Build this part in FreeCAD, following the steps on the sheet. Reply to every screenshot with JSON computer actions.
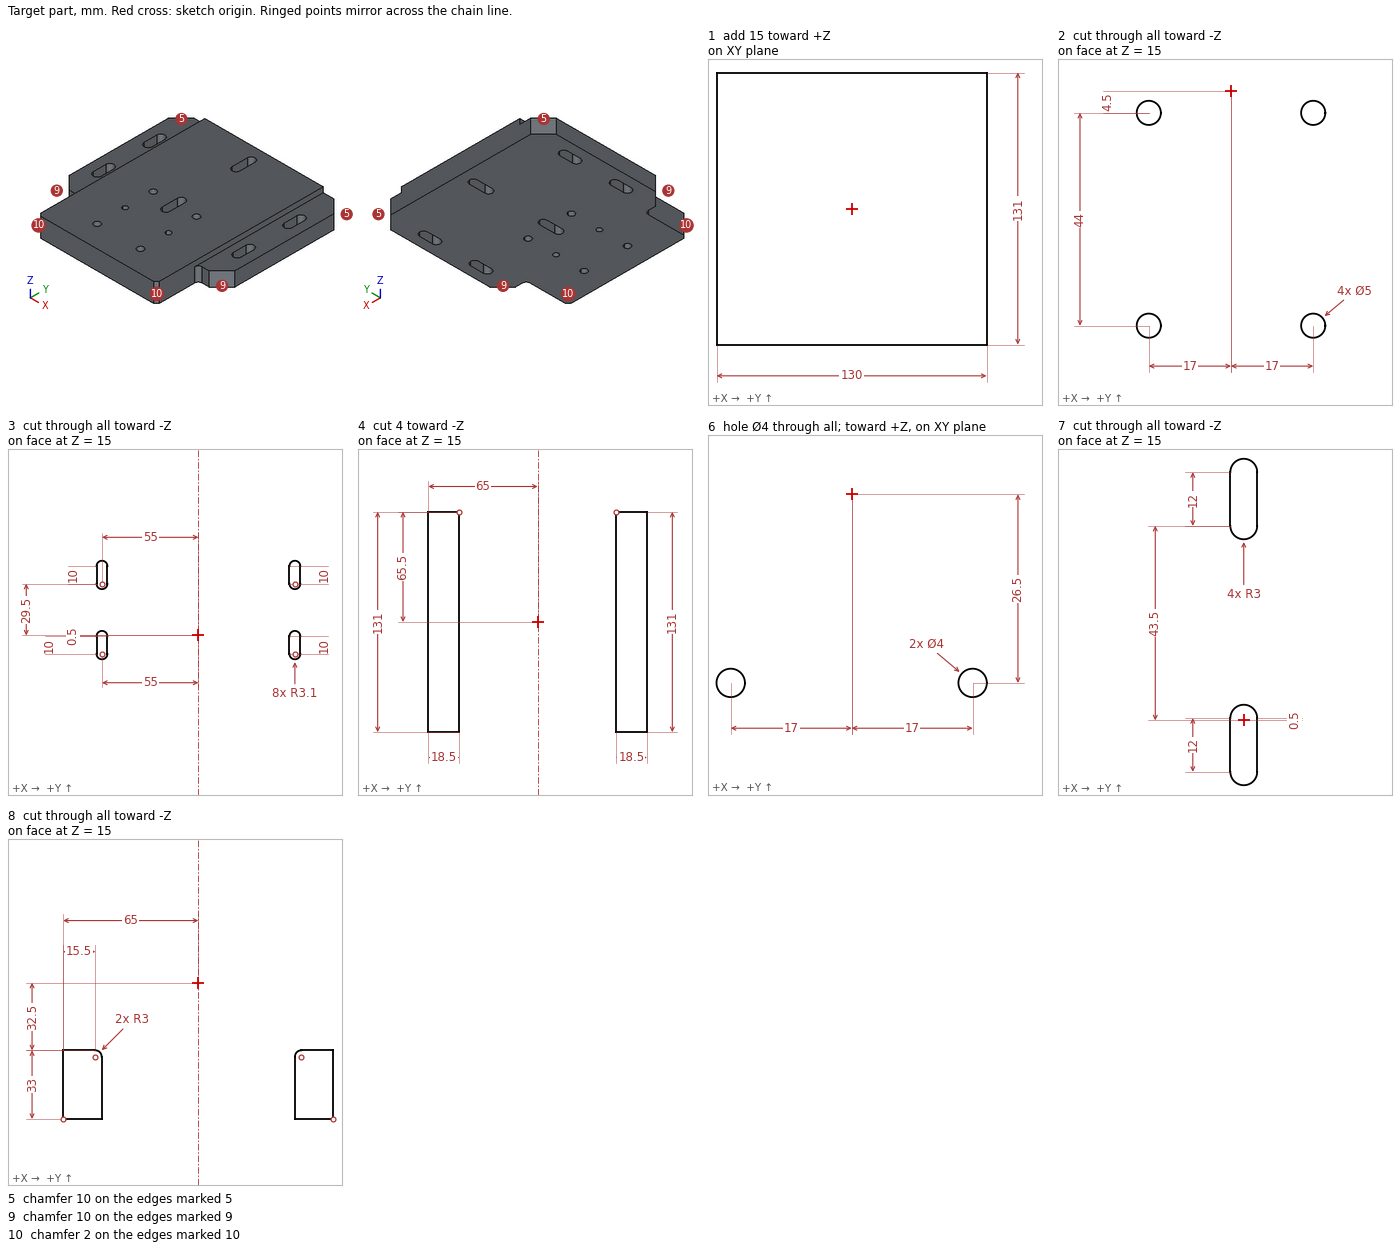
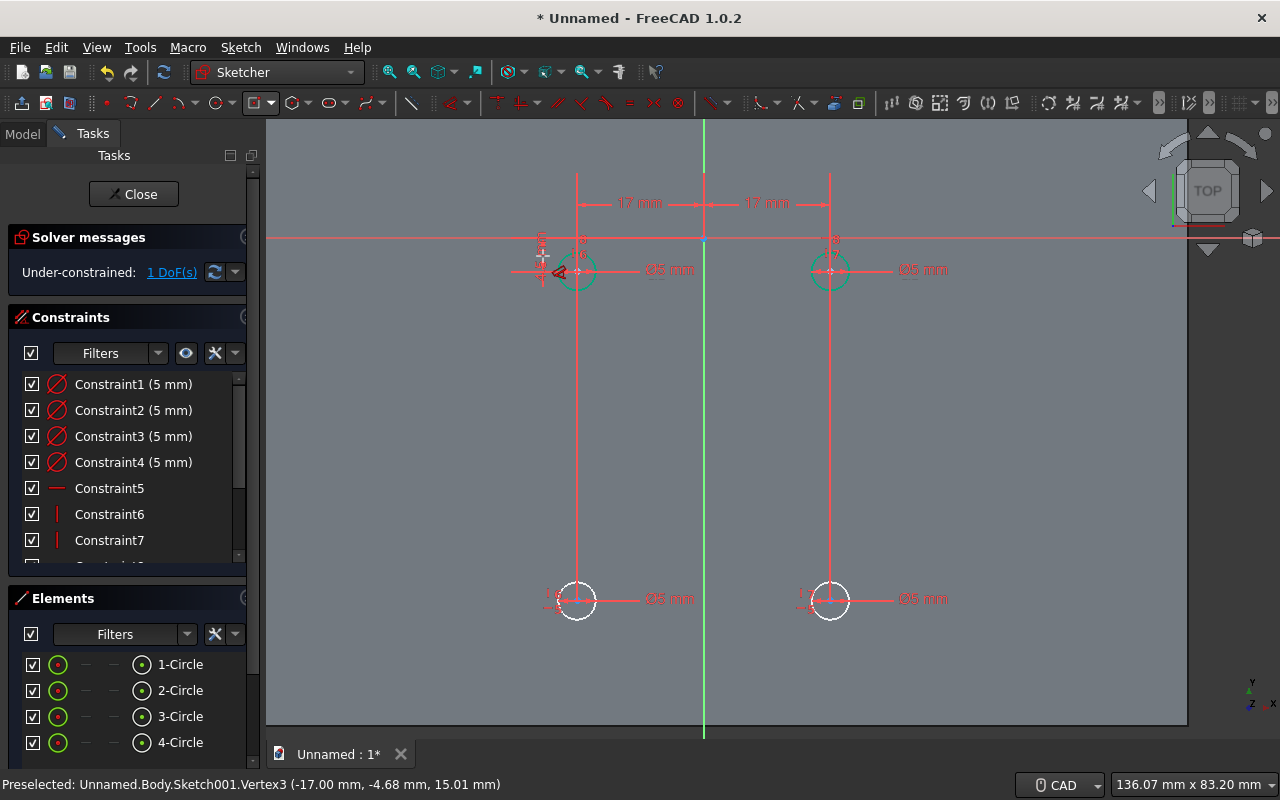
{"action": "left_click", "coordinate": [577, 601]}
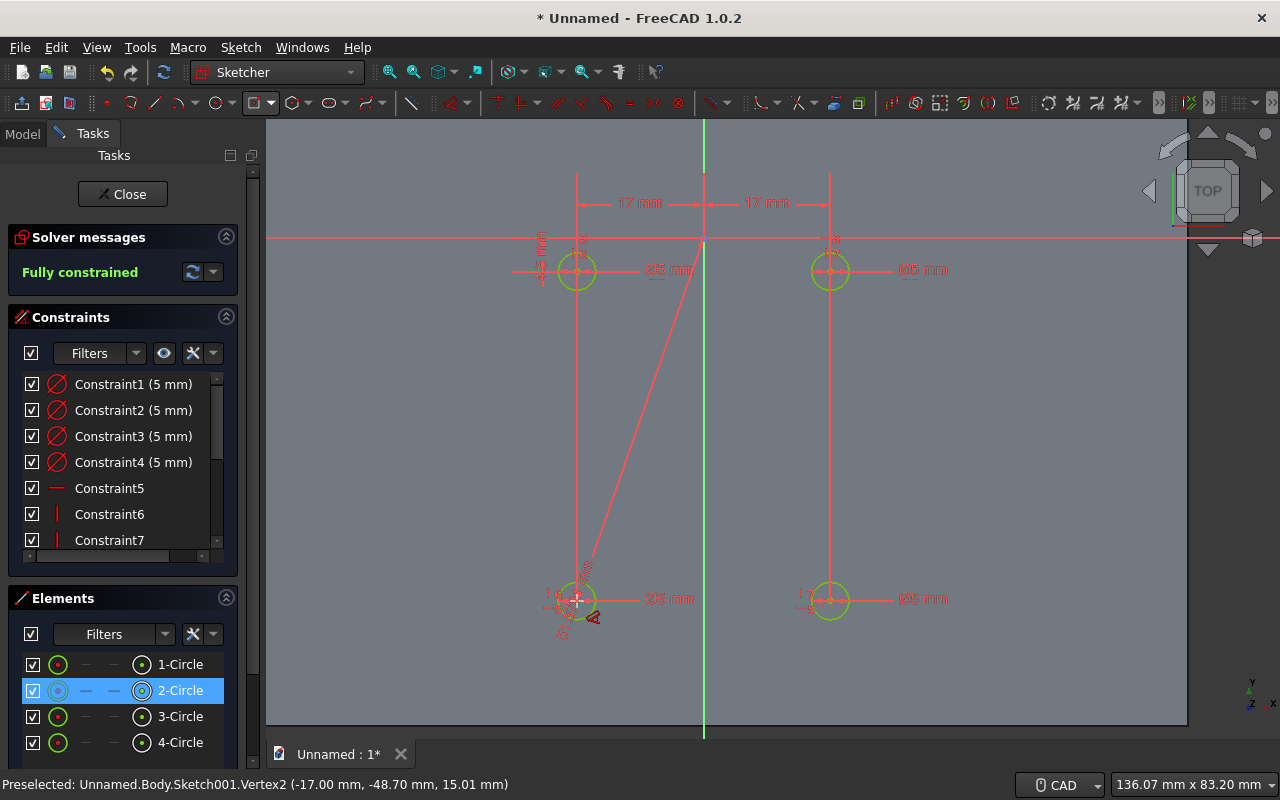
{"action": "left_click", "coordinate": [577, 272]}
{"action": "left_click", "coordinate": [543, 436]}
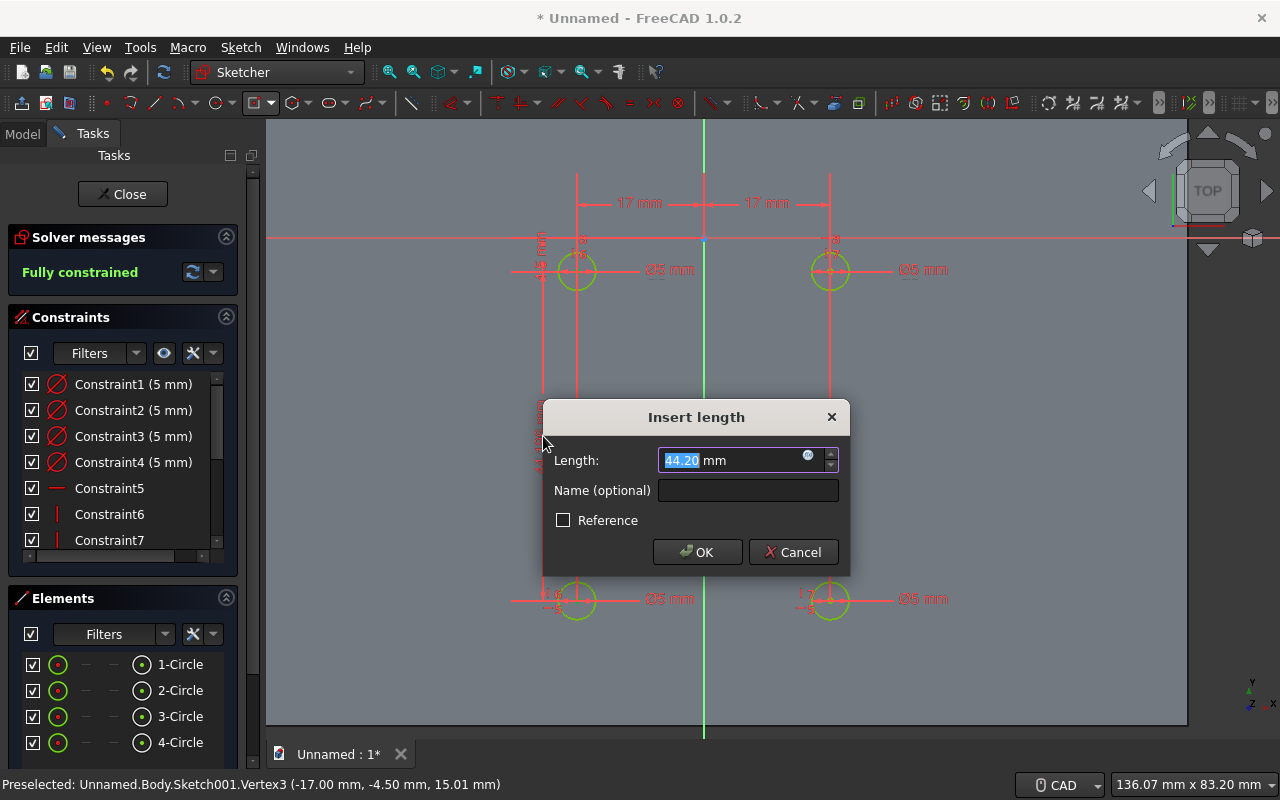
{"action": "type", "text": "44"}
{"action": "key", "text": "Return"}
{"action": "key", "text": "Escape"}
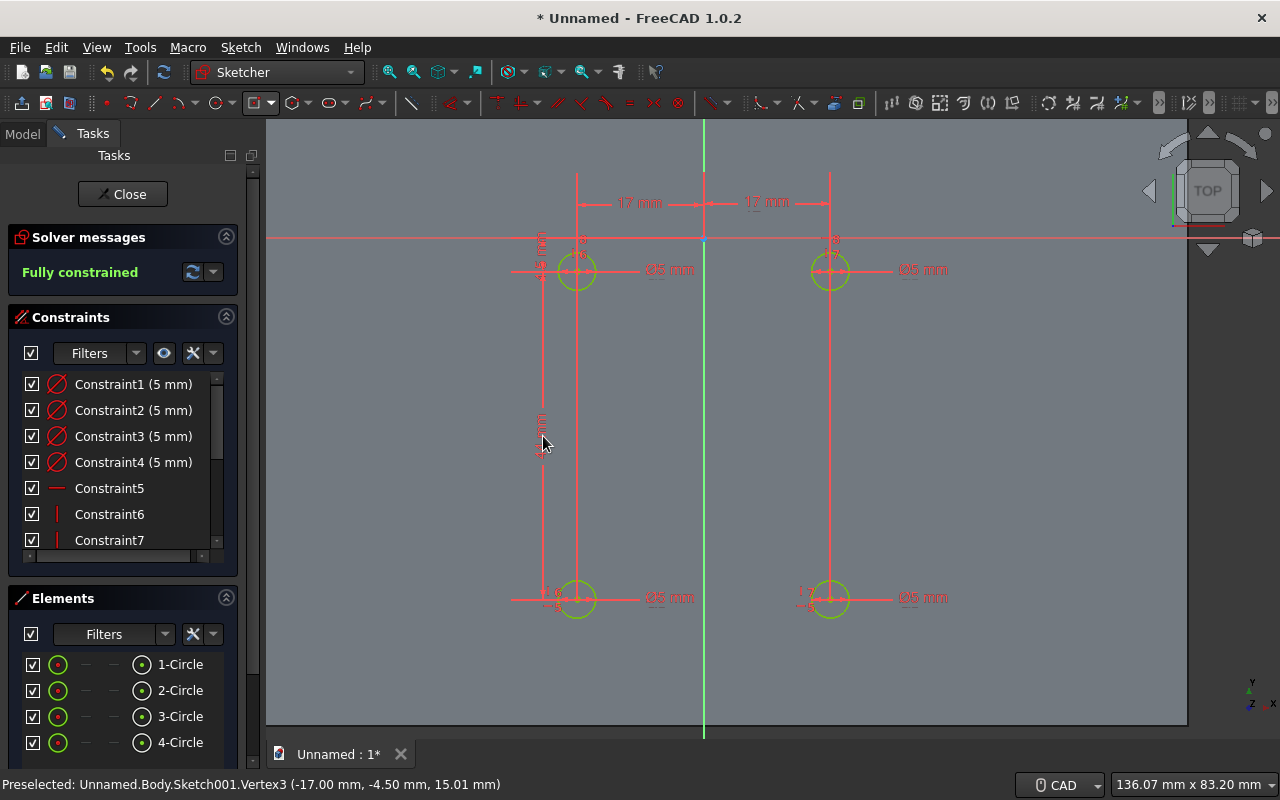
{"action": "left_click", "coordinate": [123, 194]}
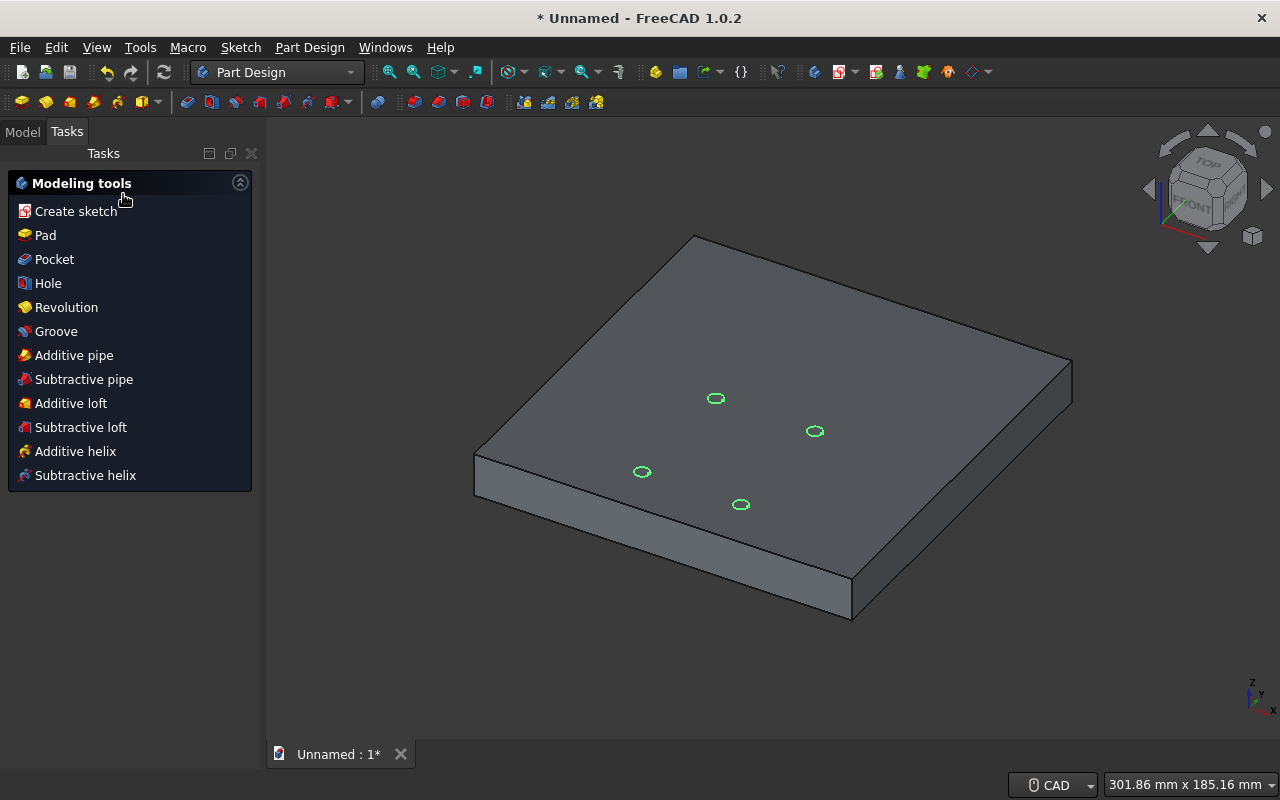
{"action": "left_click", "coordinate": [188, 102]}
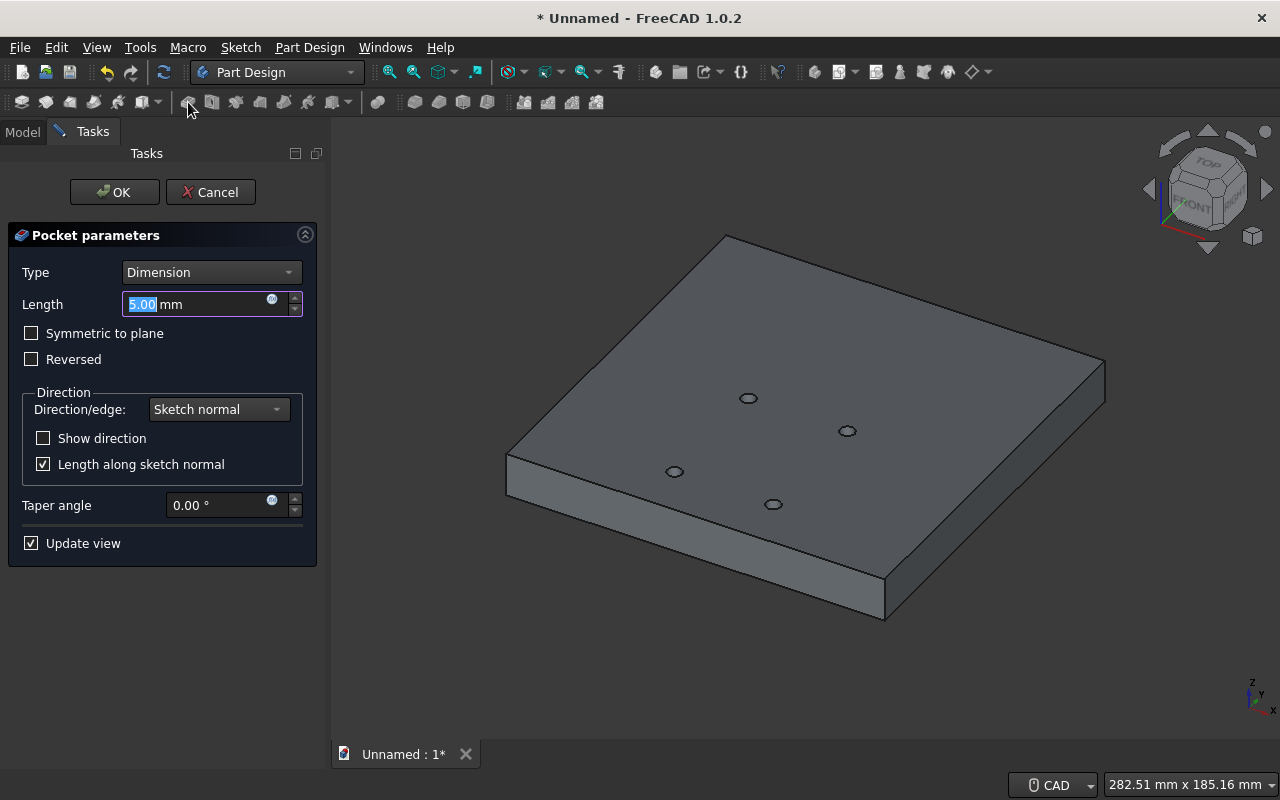
{"action": "left_click", "coordinate": [212, 272]}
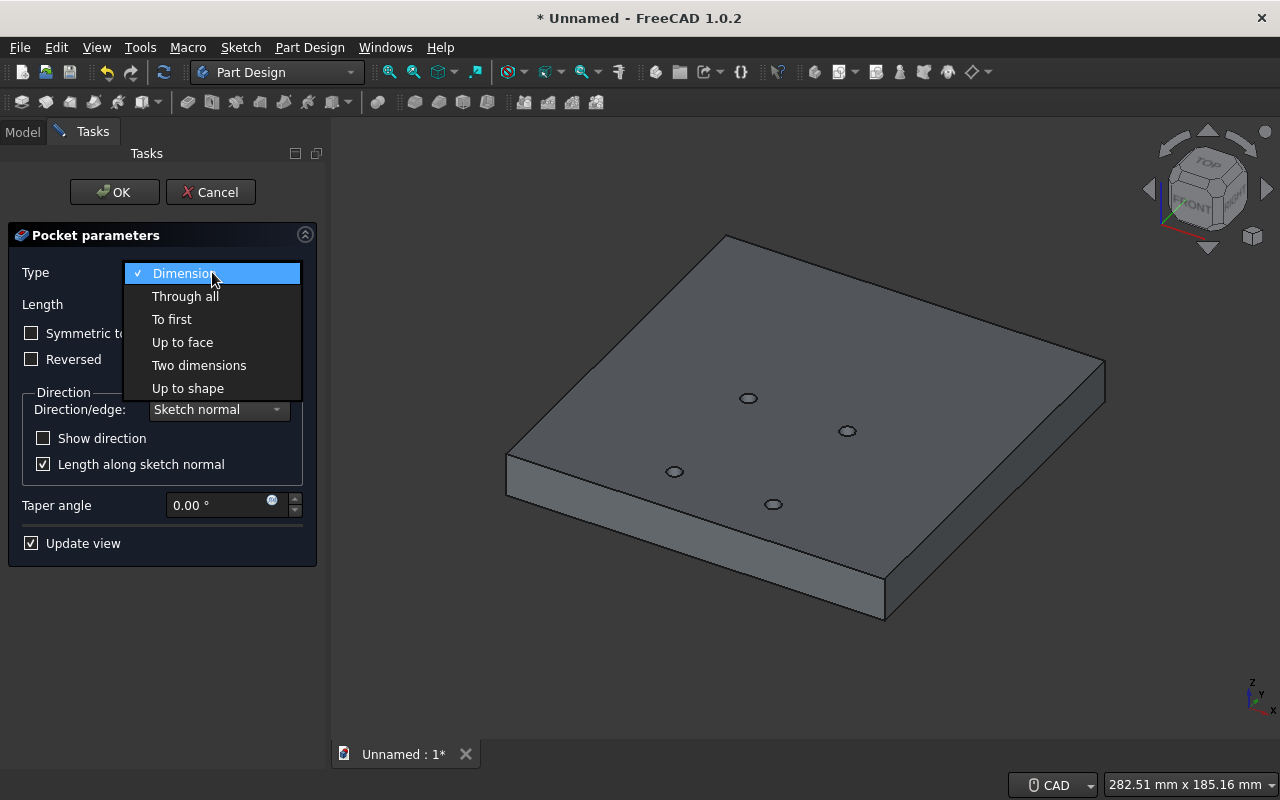
{"action": "left_click", "coordinate": [212, 296]}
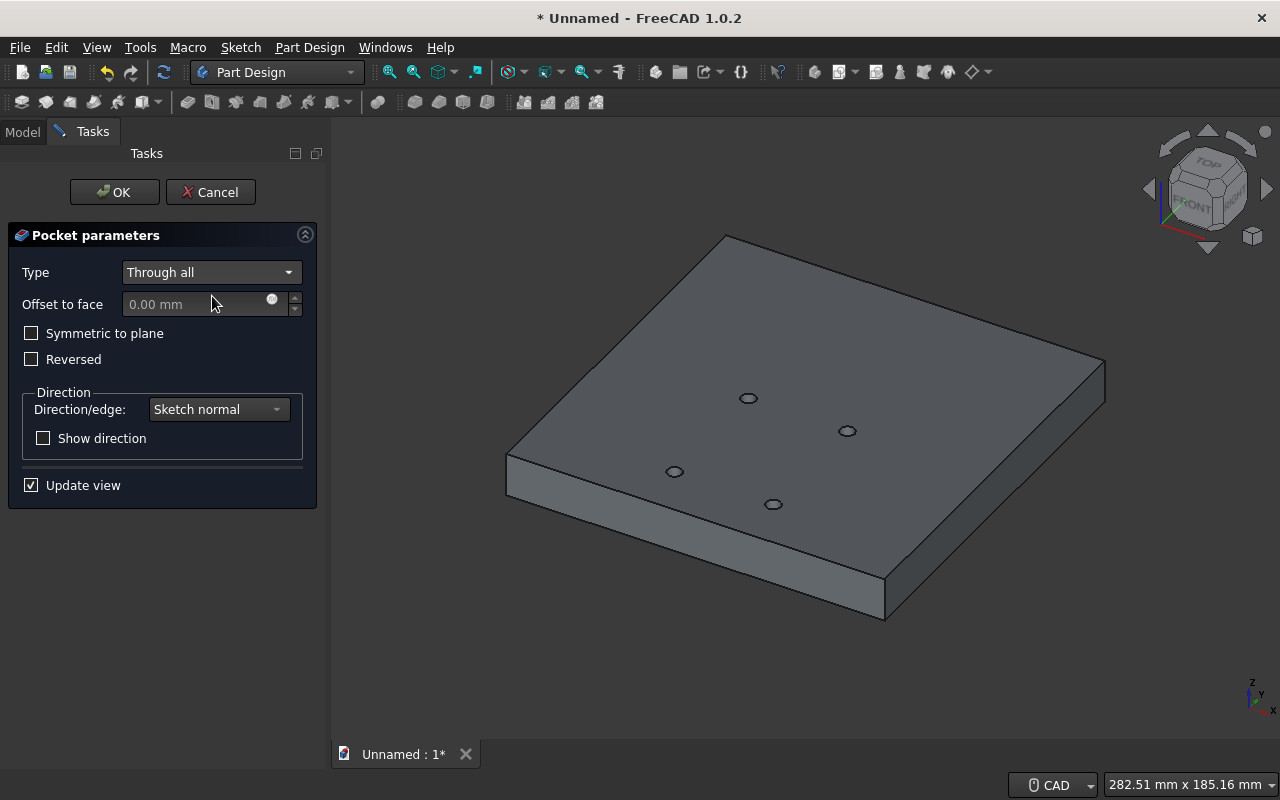
{"action": "left_click", "coordinate": [115, 192]}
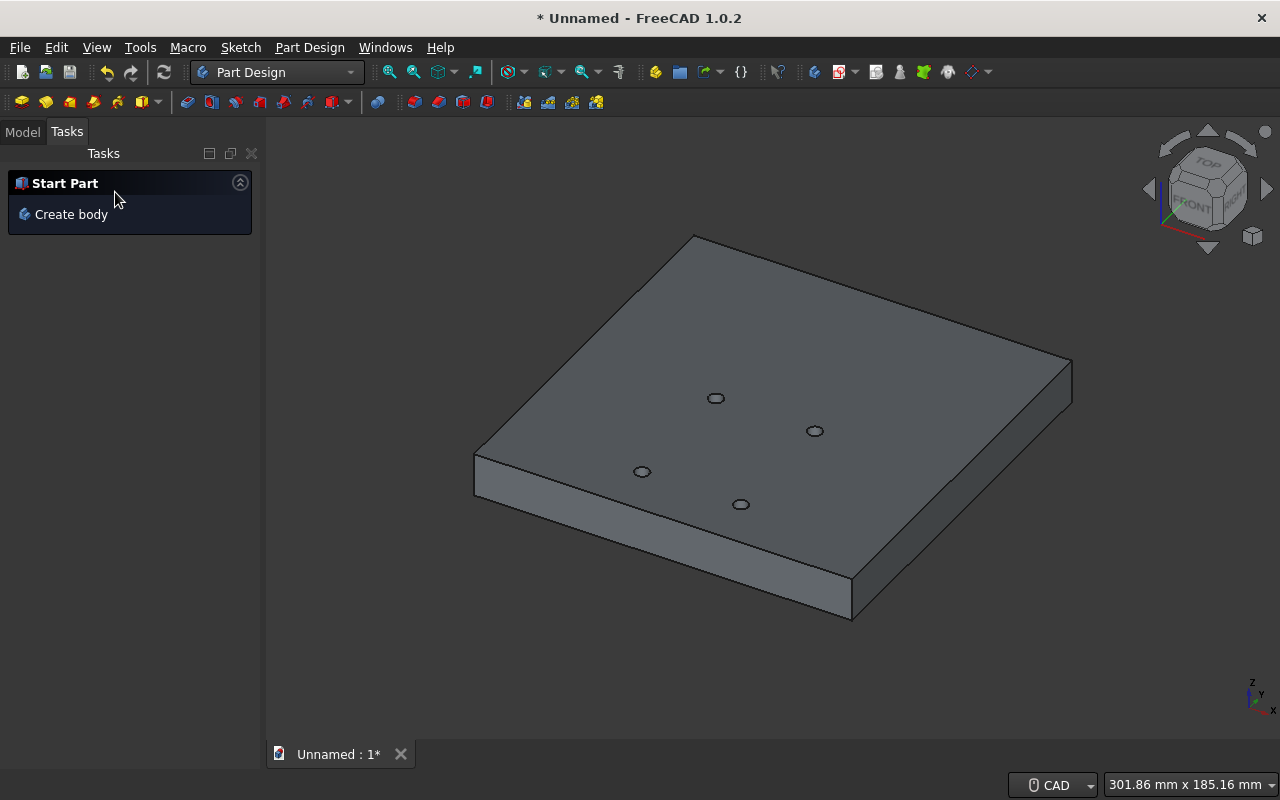
{"action": "left_click", "coordinate": [890, 362]}